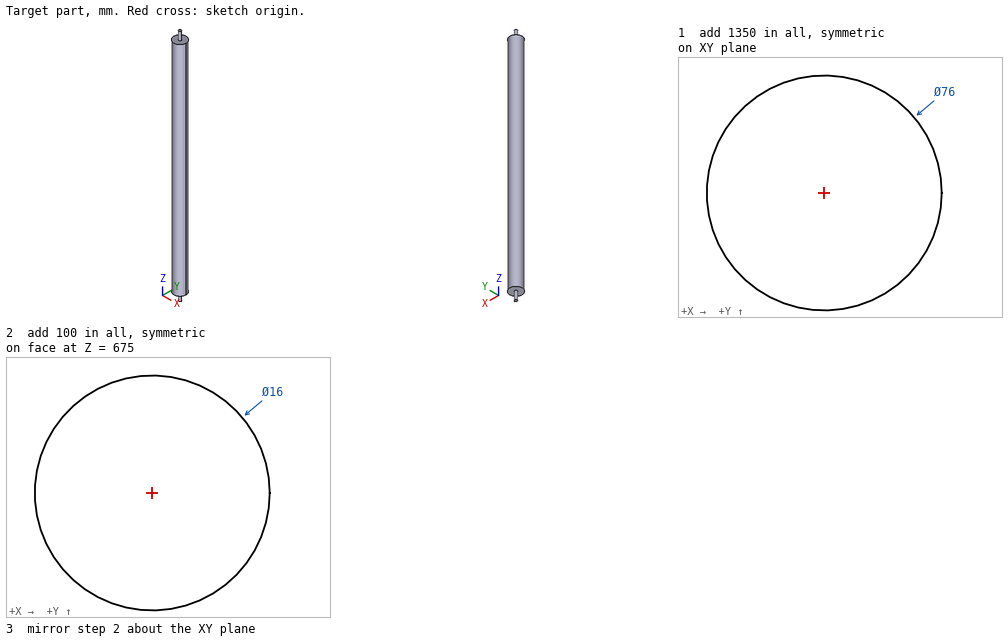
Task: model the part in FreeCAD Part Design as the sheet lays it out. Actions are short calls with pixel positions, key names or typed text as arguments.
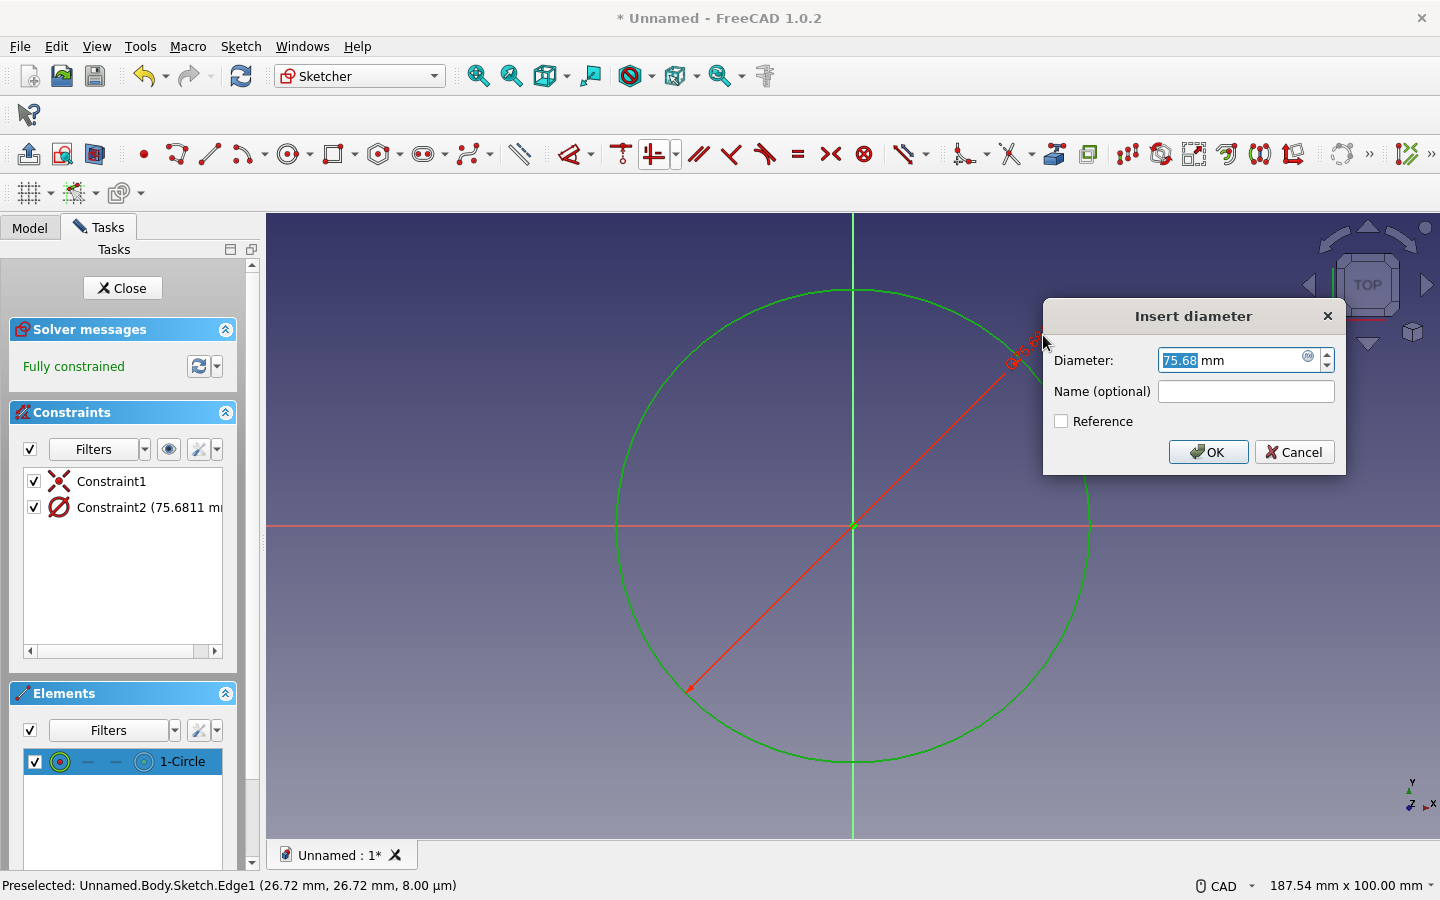
text(76)
key(Return)
key(Escape)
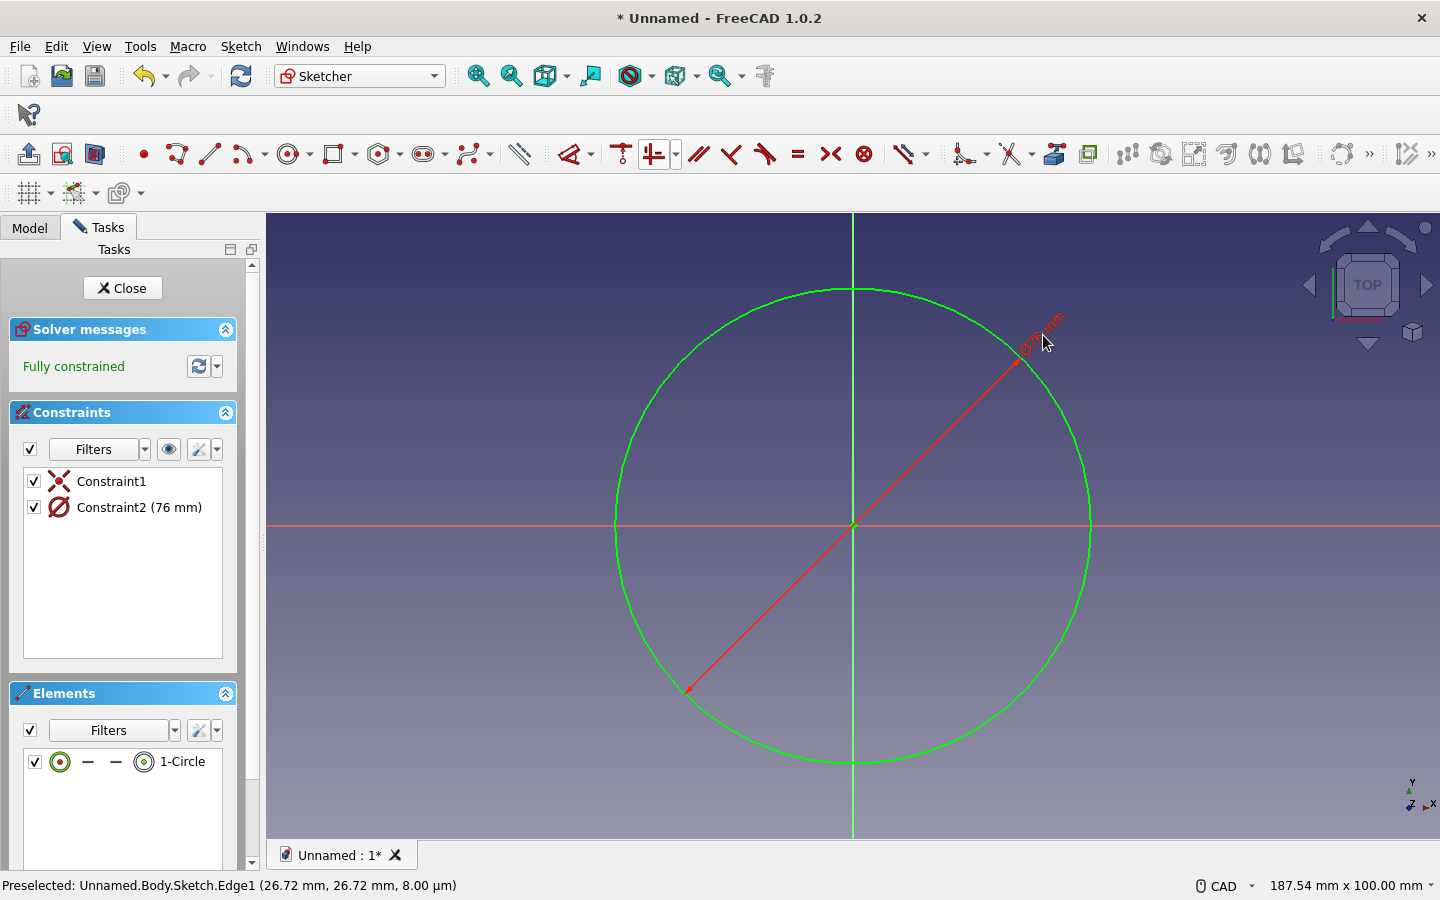
click(123, 288)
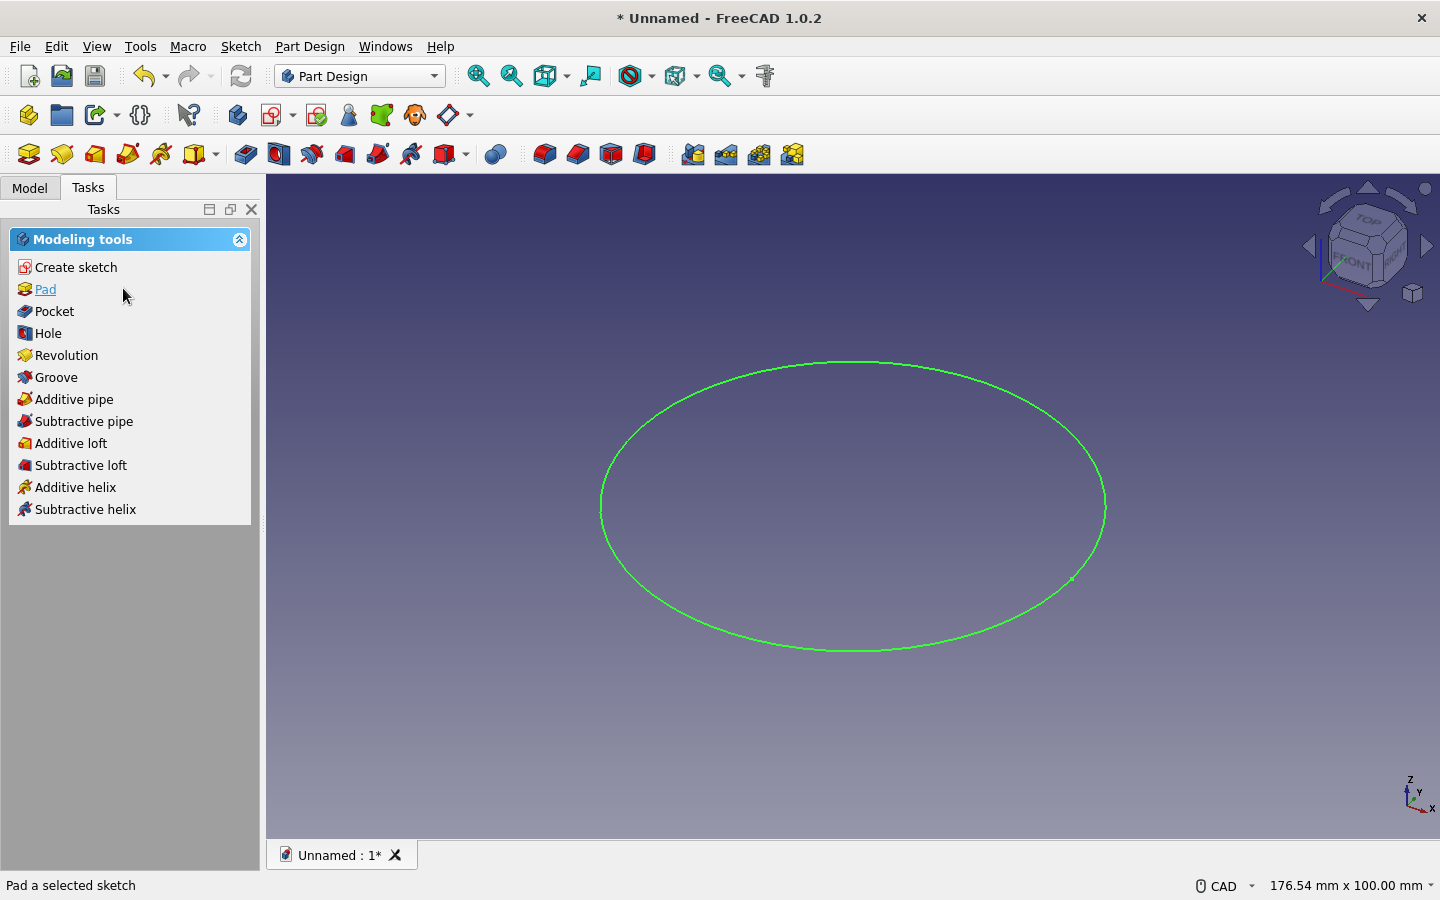
click(29, 154)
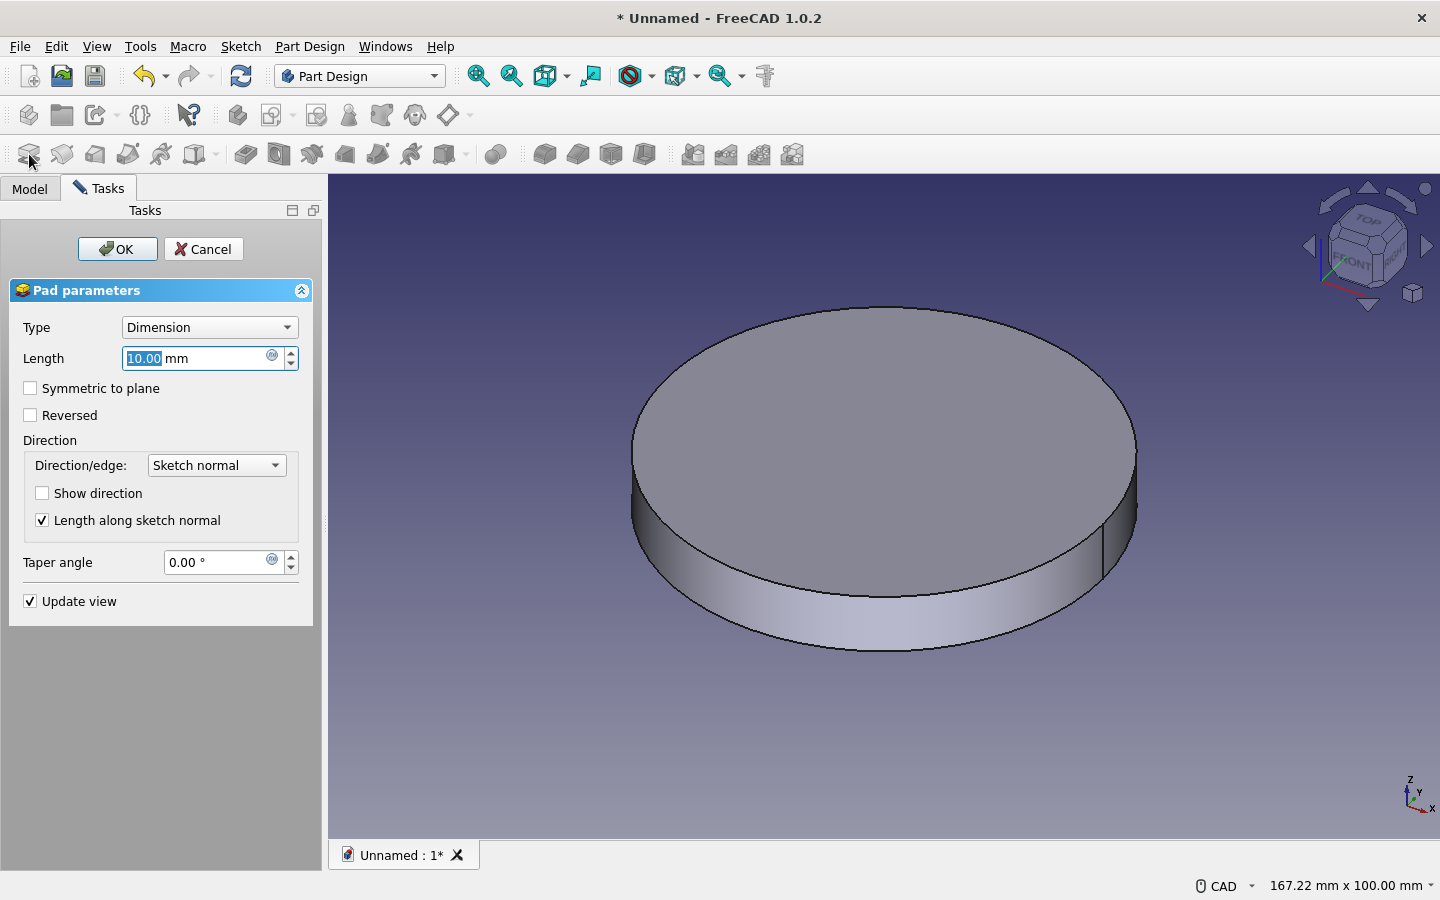
text(1350)
key(Tab)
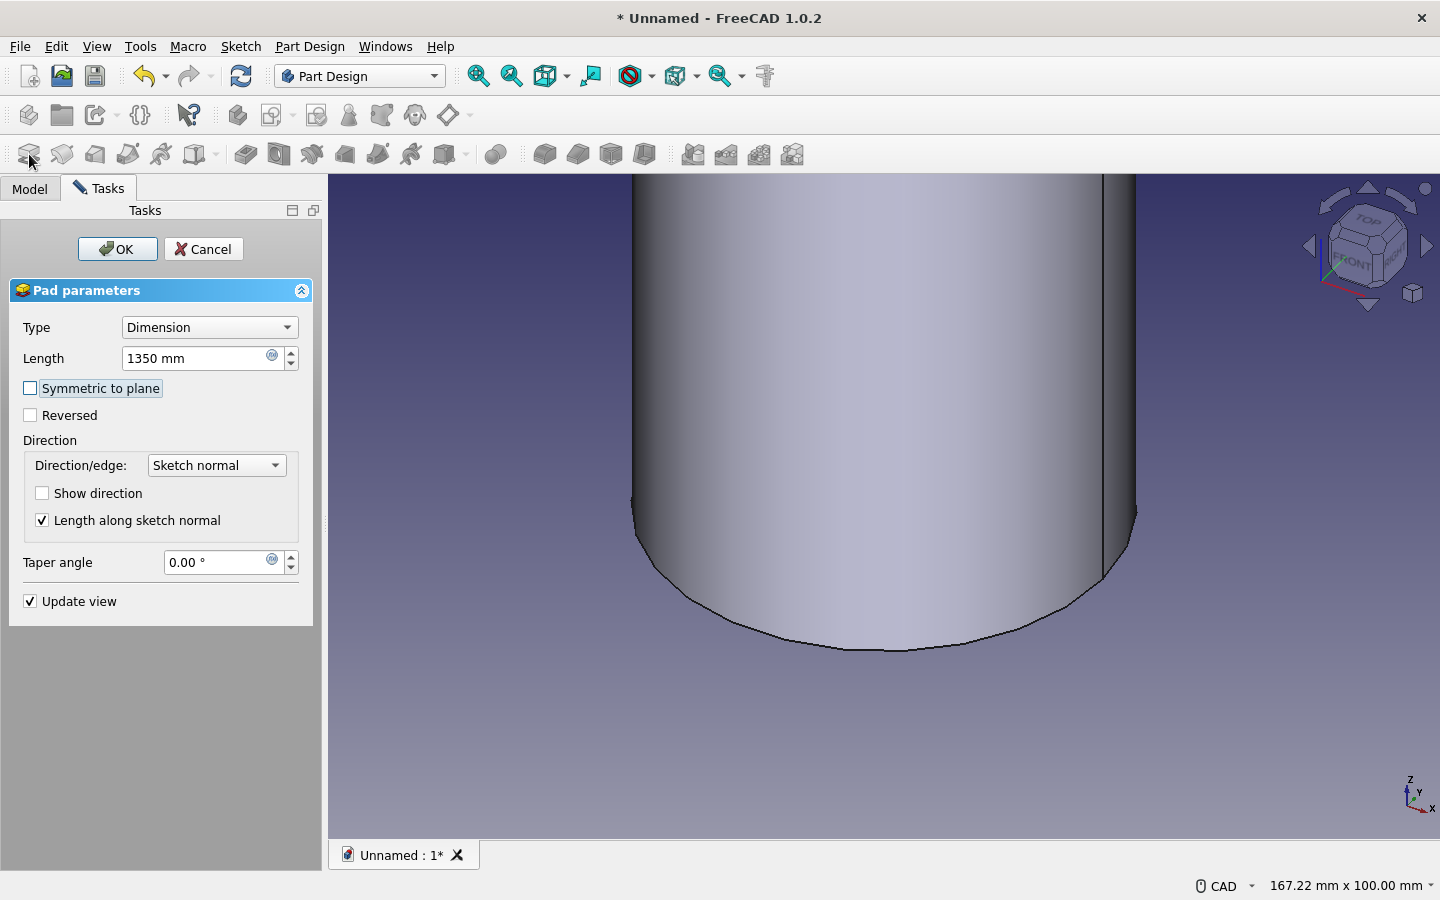
click(31, 388)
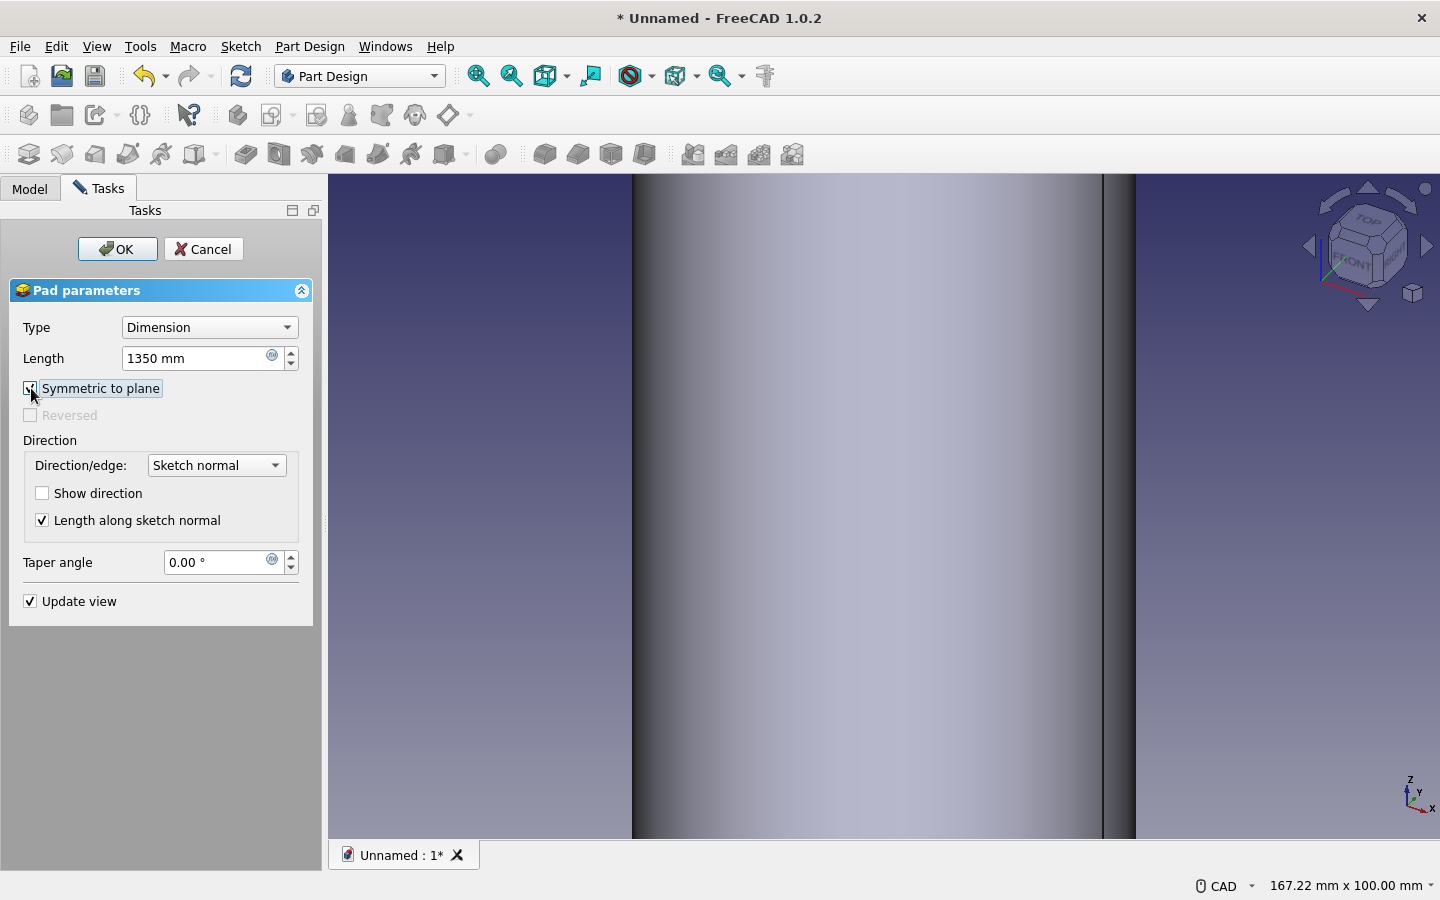
click(118, 249)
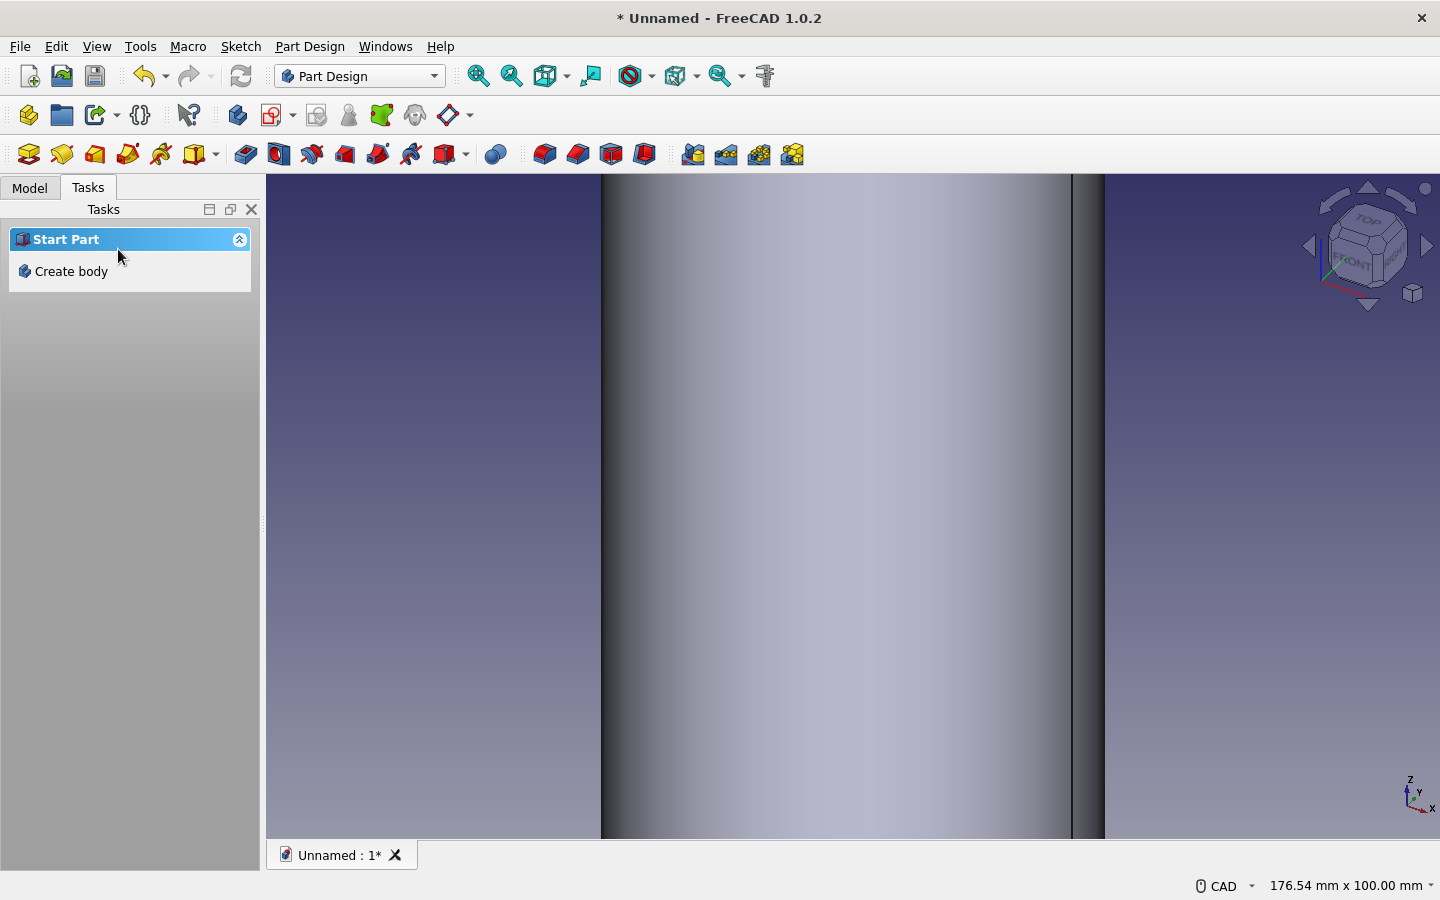
click(479, 76)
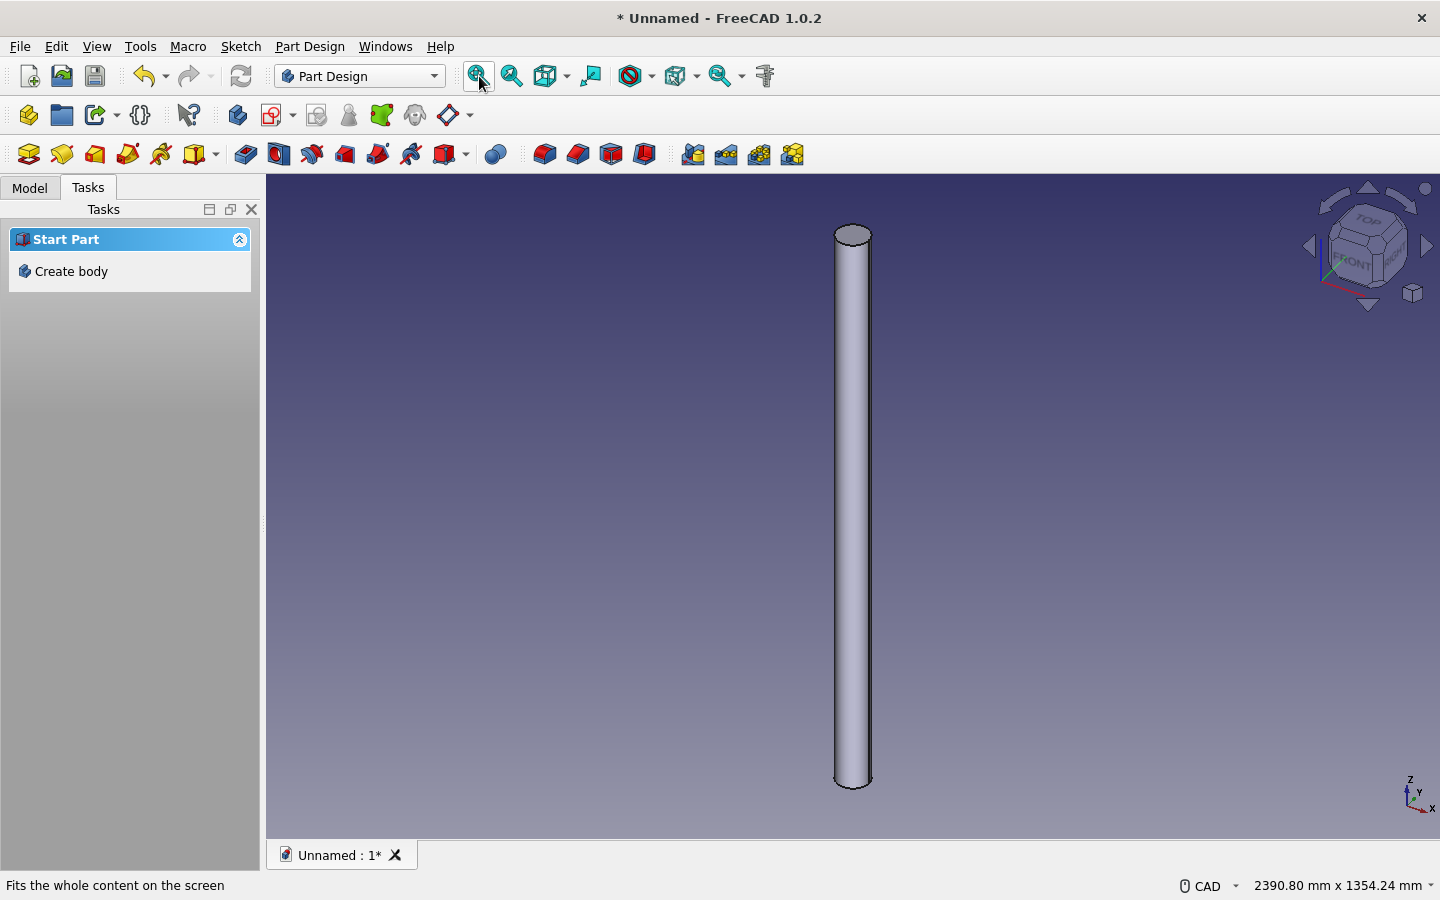
click(853, 234)